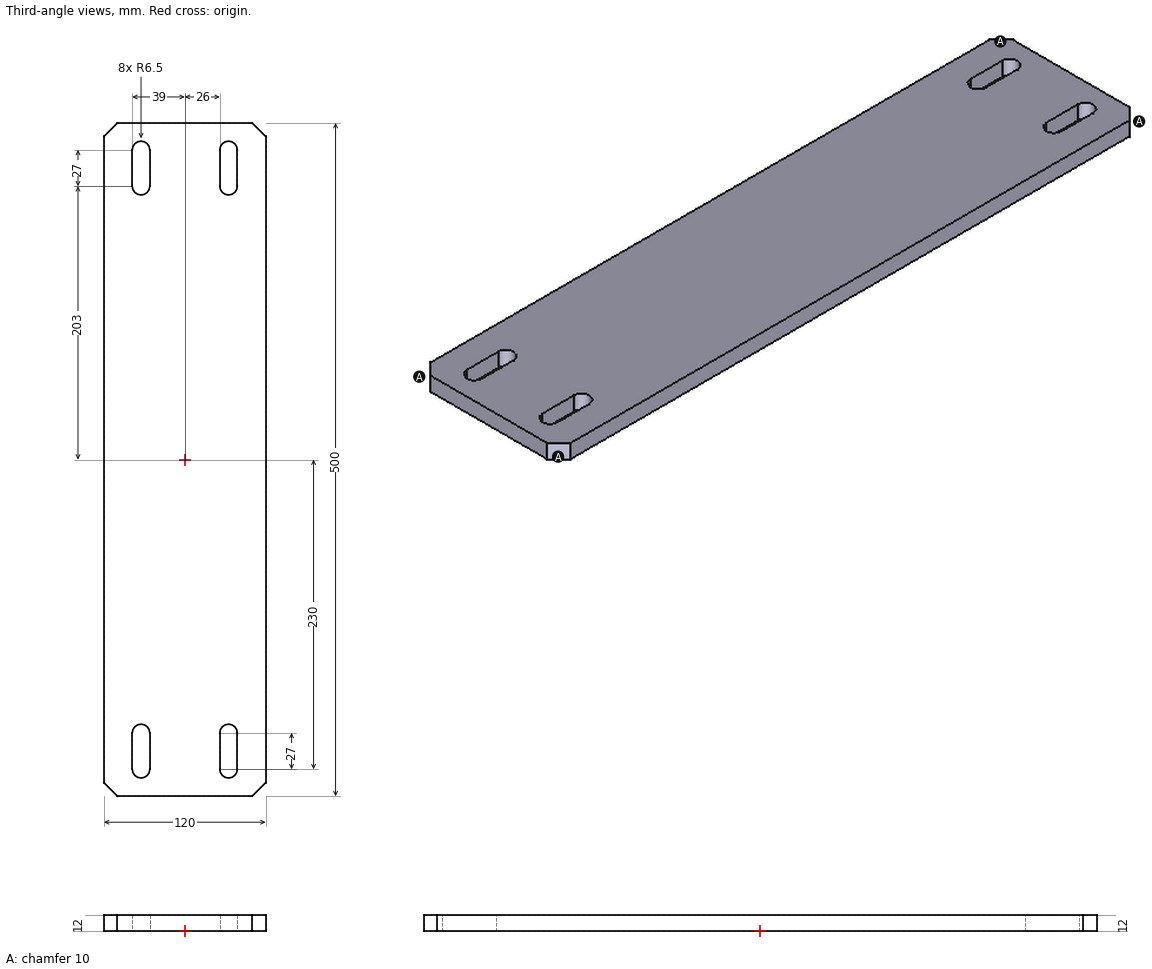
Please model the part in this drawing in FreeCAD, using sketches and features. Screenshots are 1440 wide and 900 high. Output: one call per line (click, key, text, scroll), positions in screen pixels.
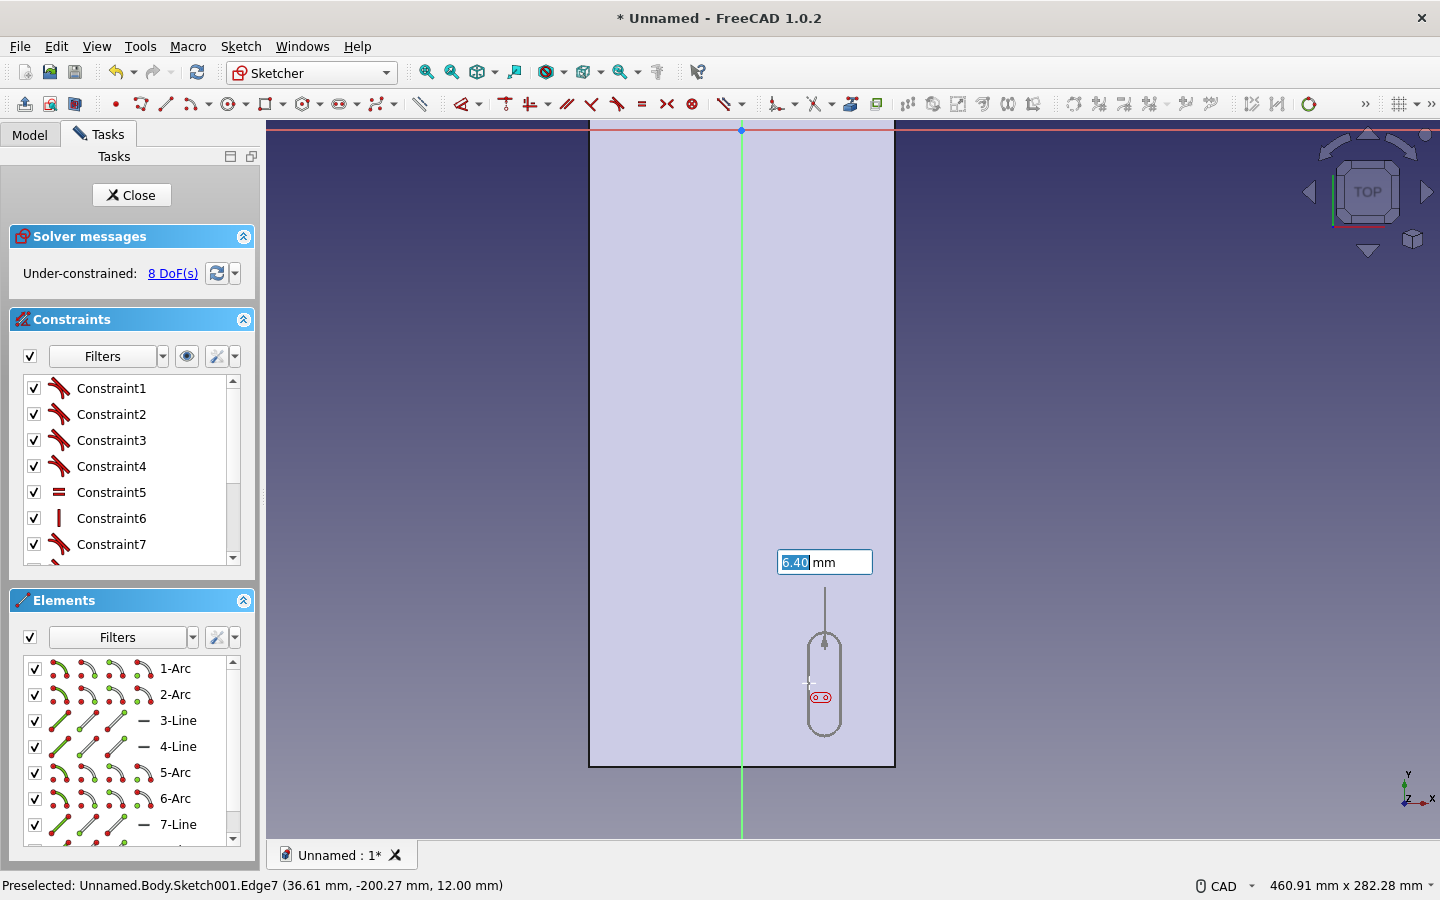
click(808, 682)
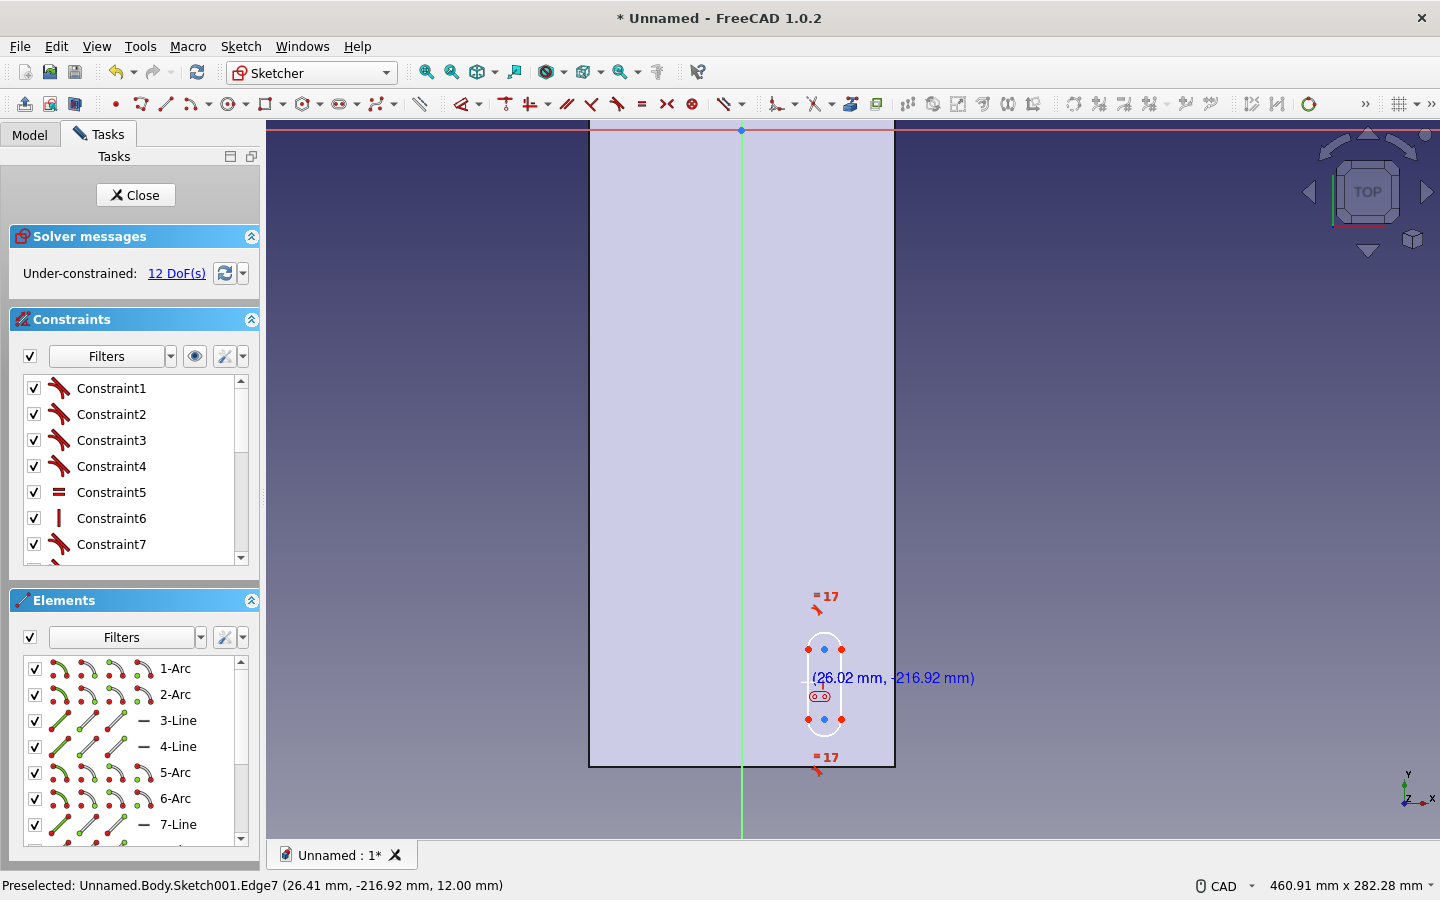
scroll(659, 716, up, 2)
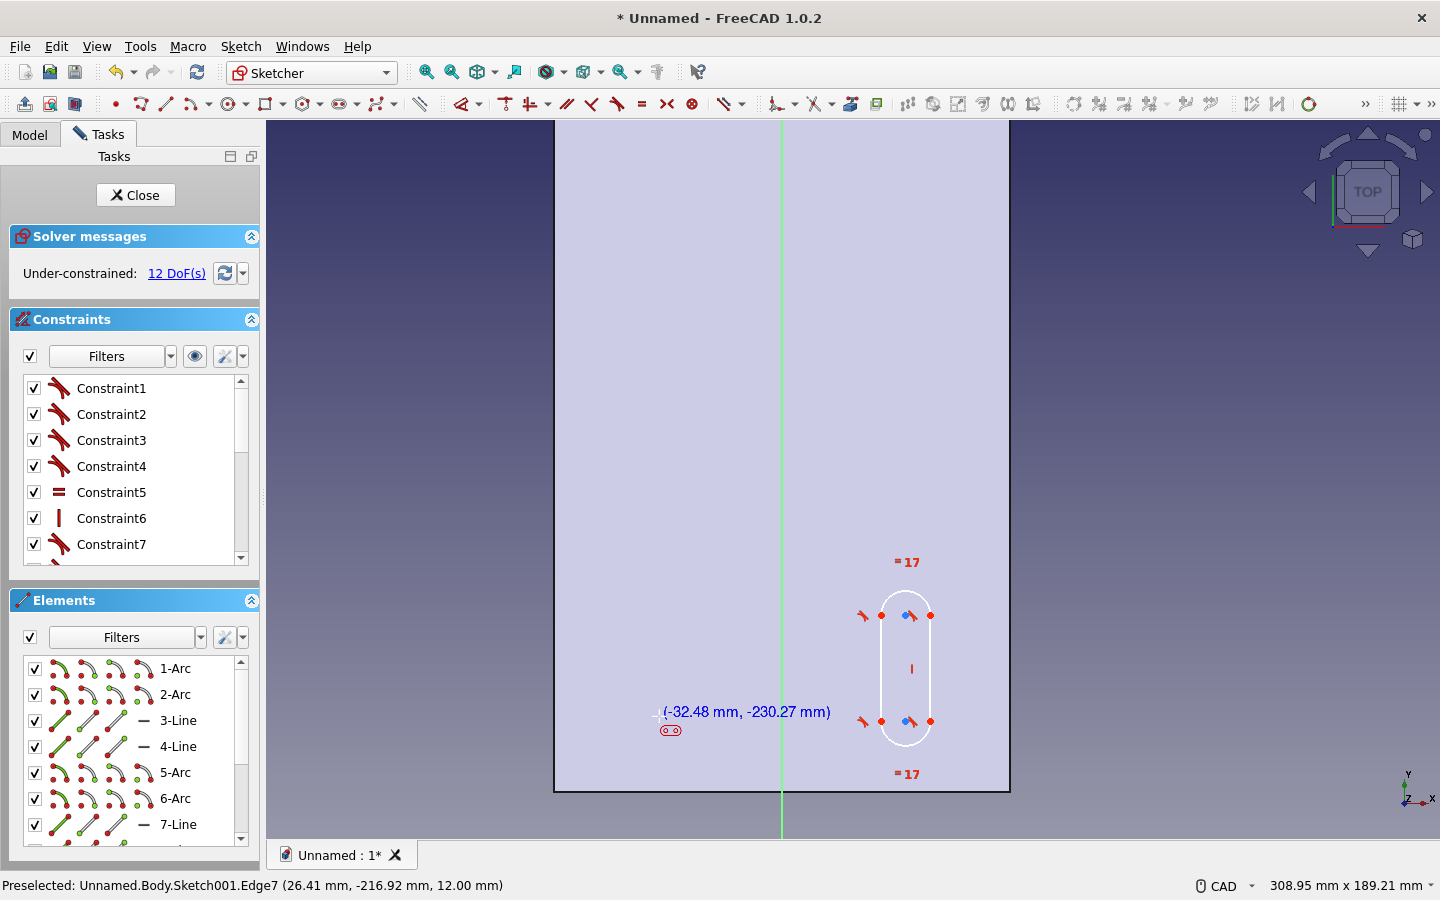
scroll(785, 688, down, 7)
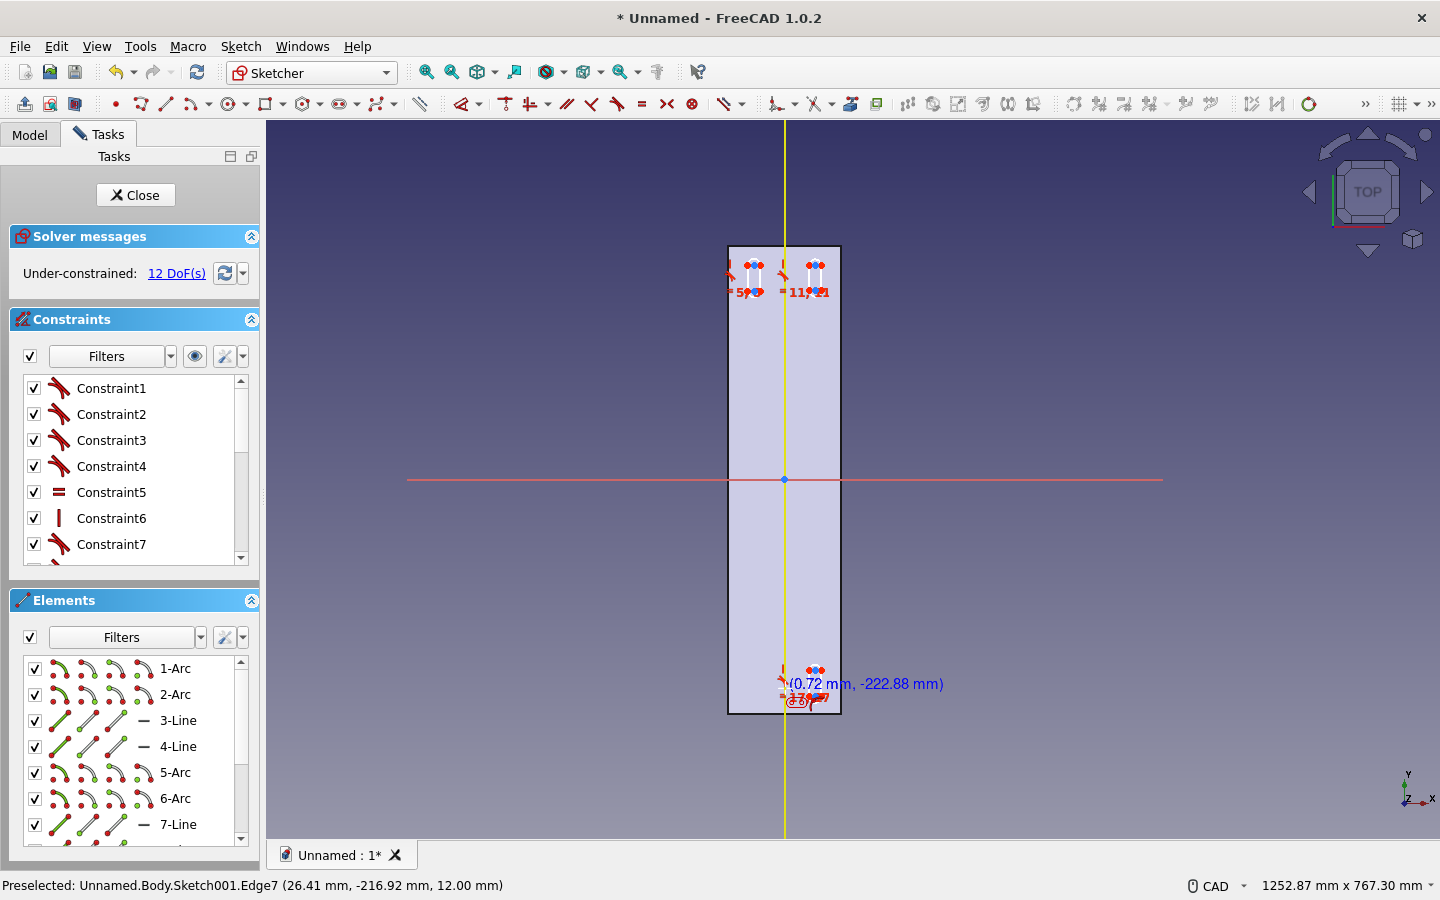
click(754, 696)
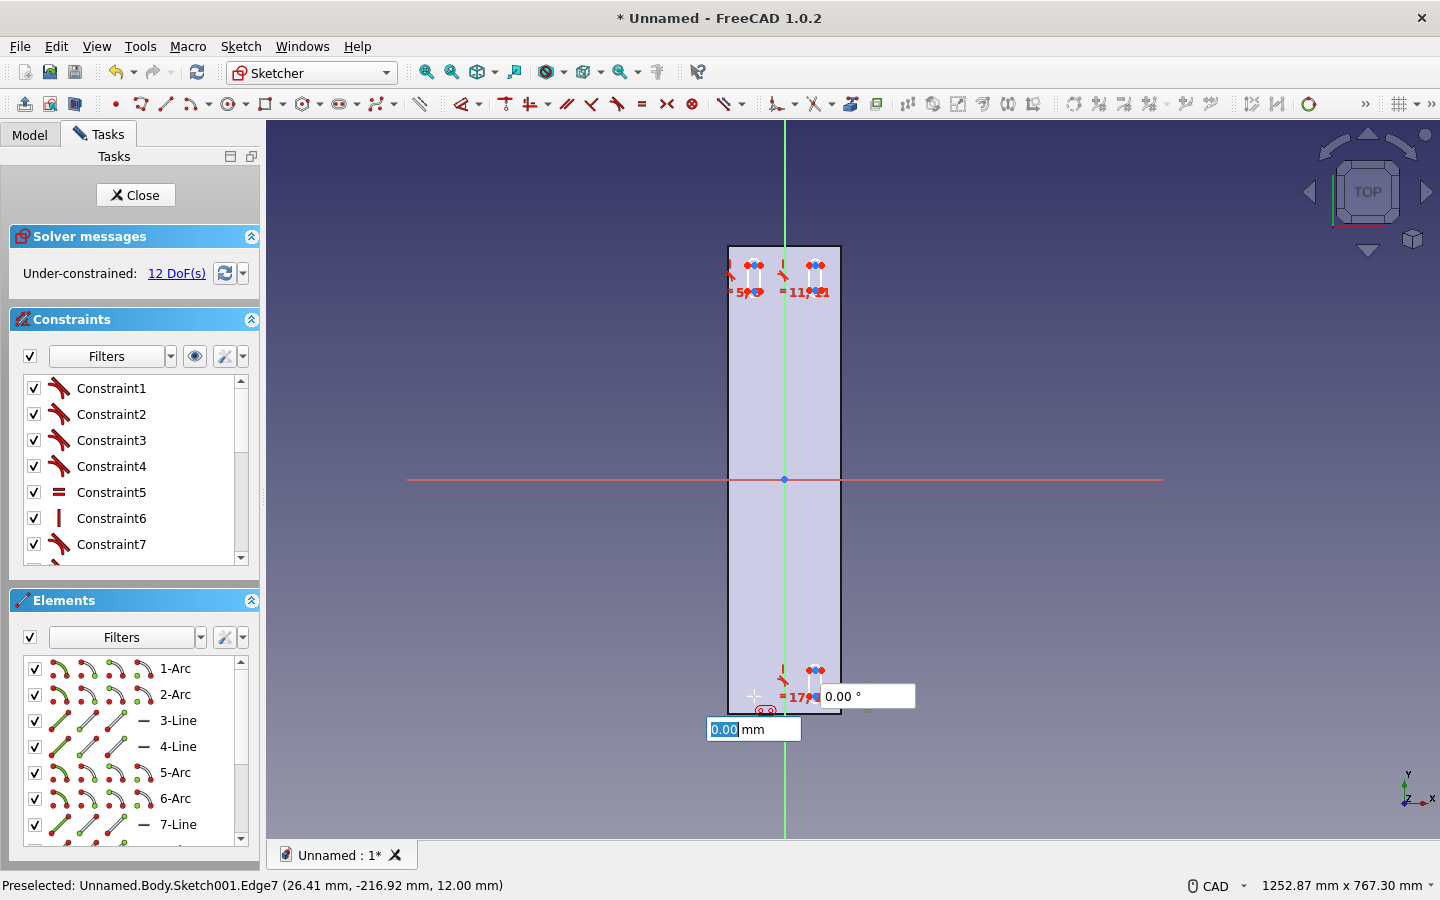
click(754, 670)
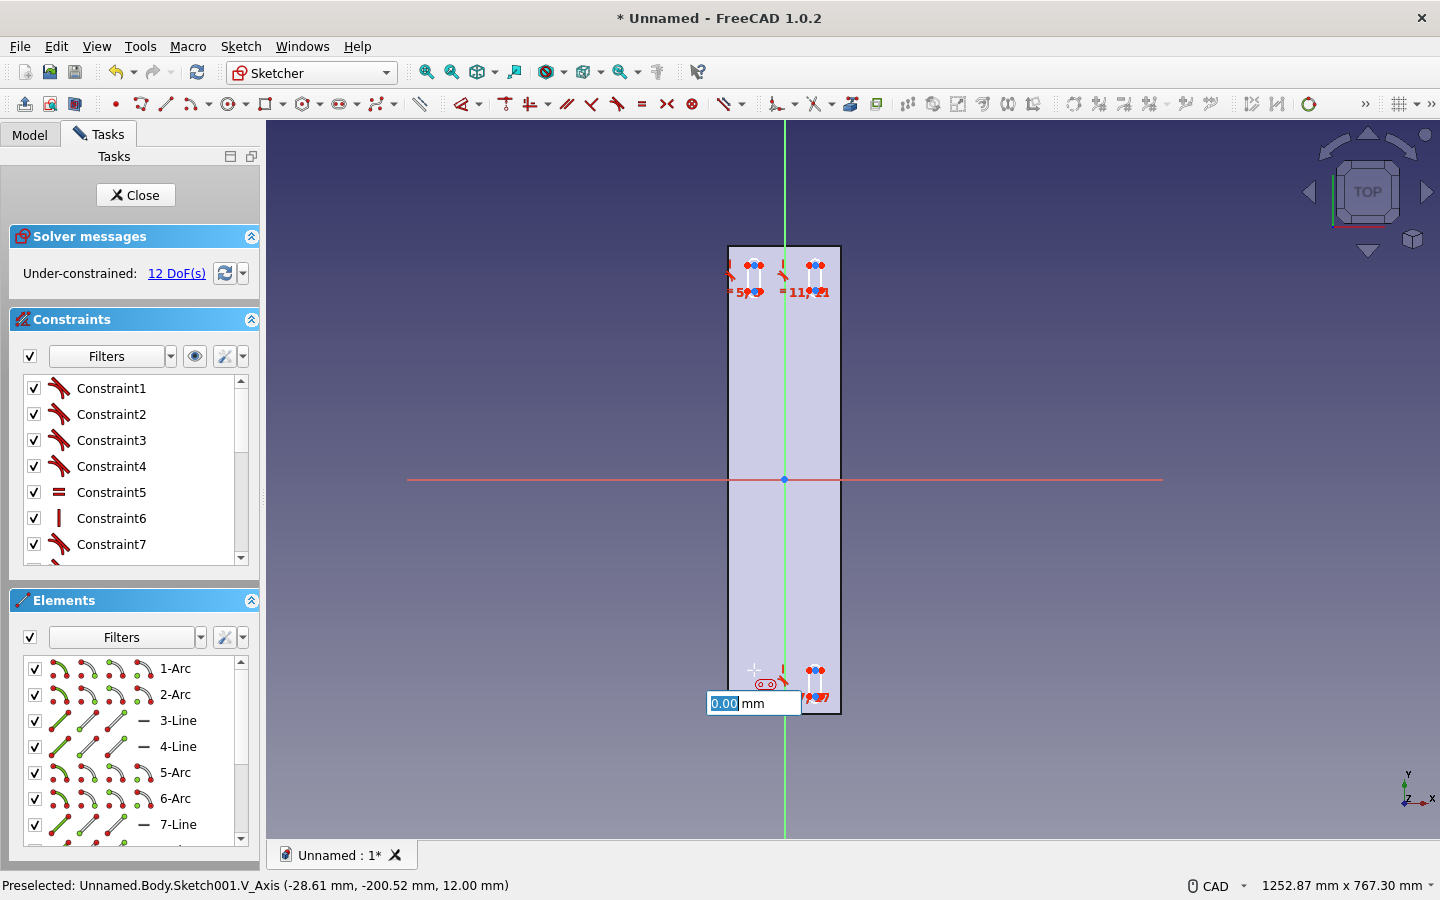
scroll(760, 683, up, 5)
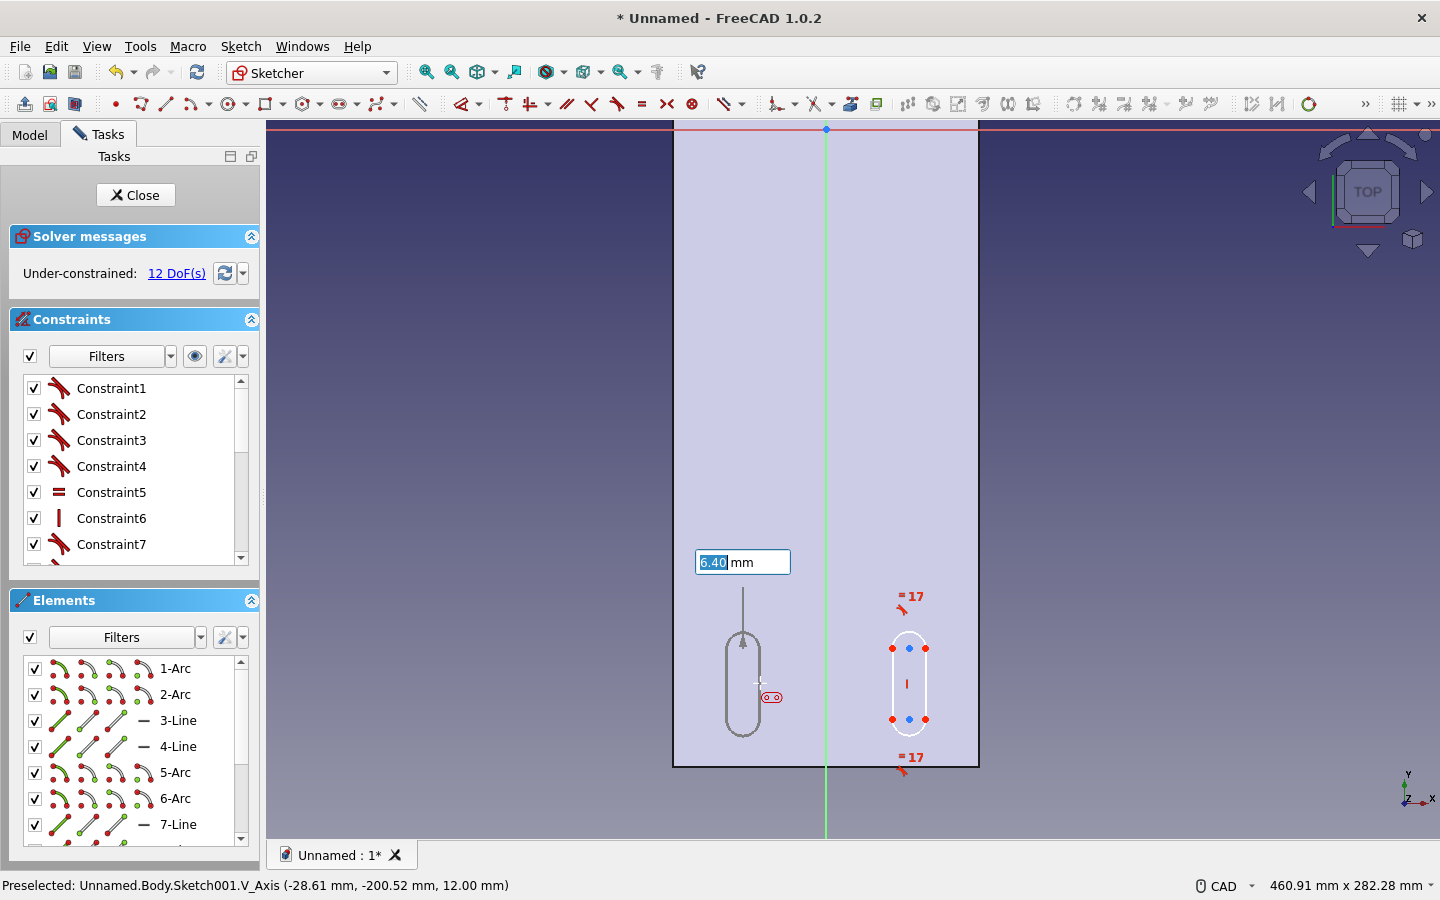
click(760, 681)
key(Escape)